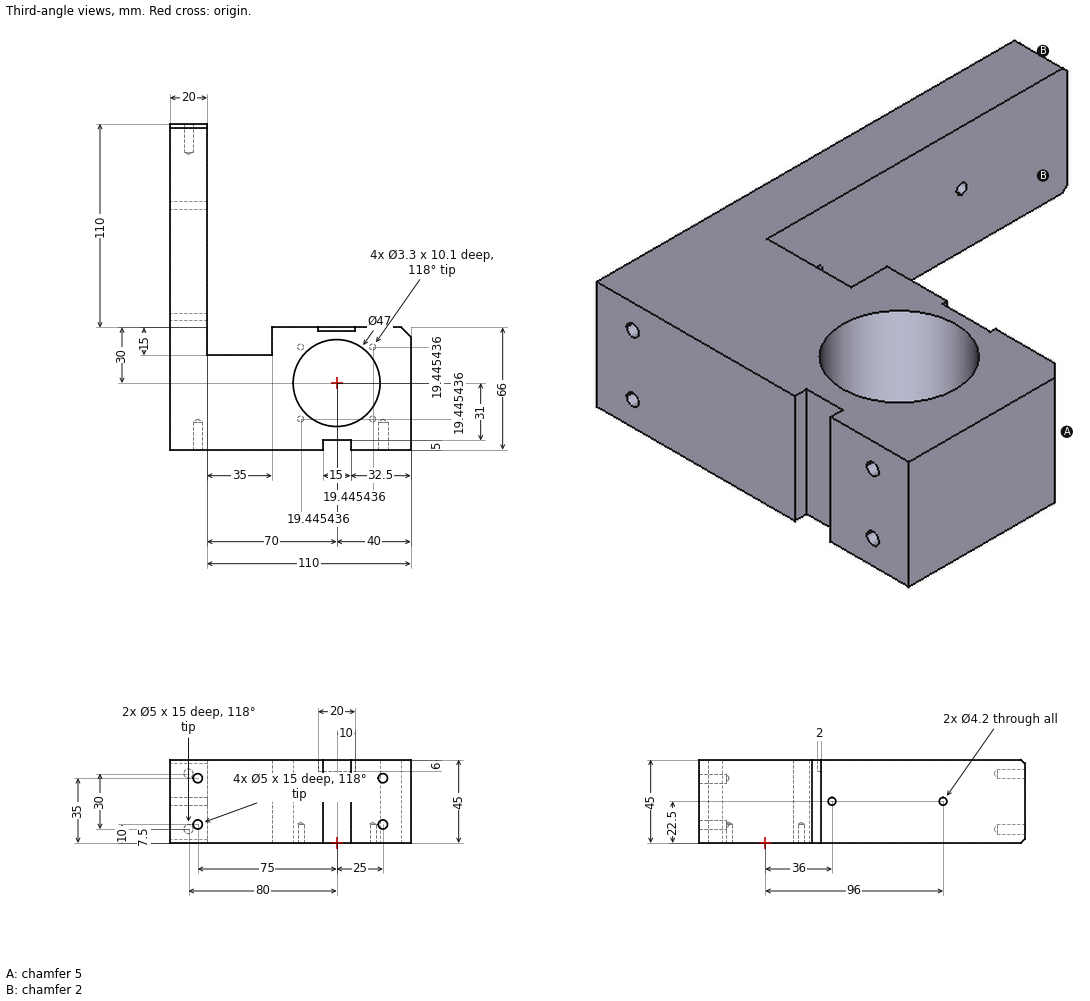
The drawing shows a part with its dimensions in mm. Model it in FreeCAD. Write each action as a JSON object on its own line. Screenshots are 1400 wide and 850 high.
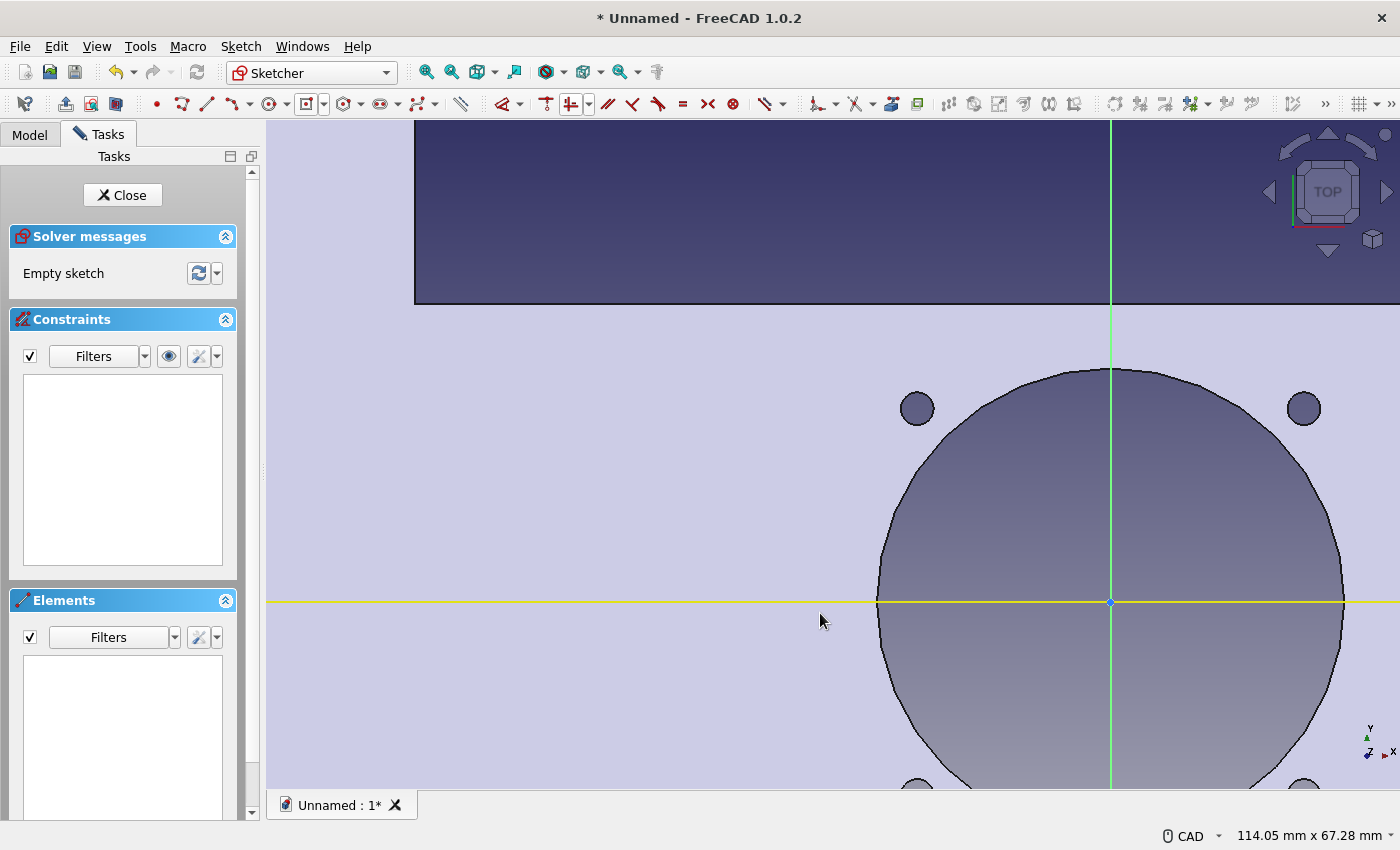
{"action": "left_click", "coordinate": [324, 104]}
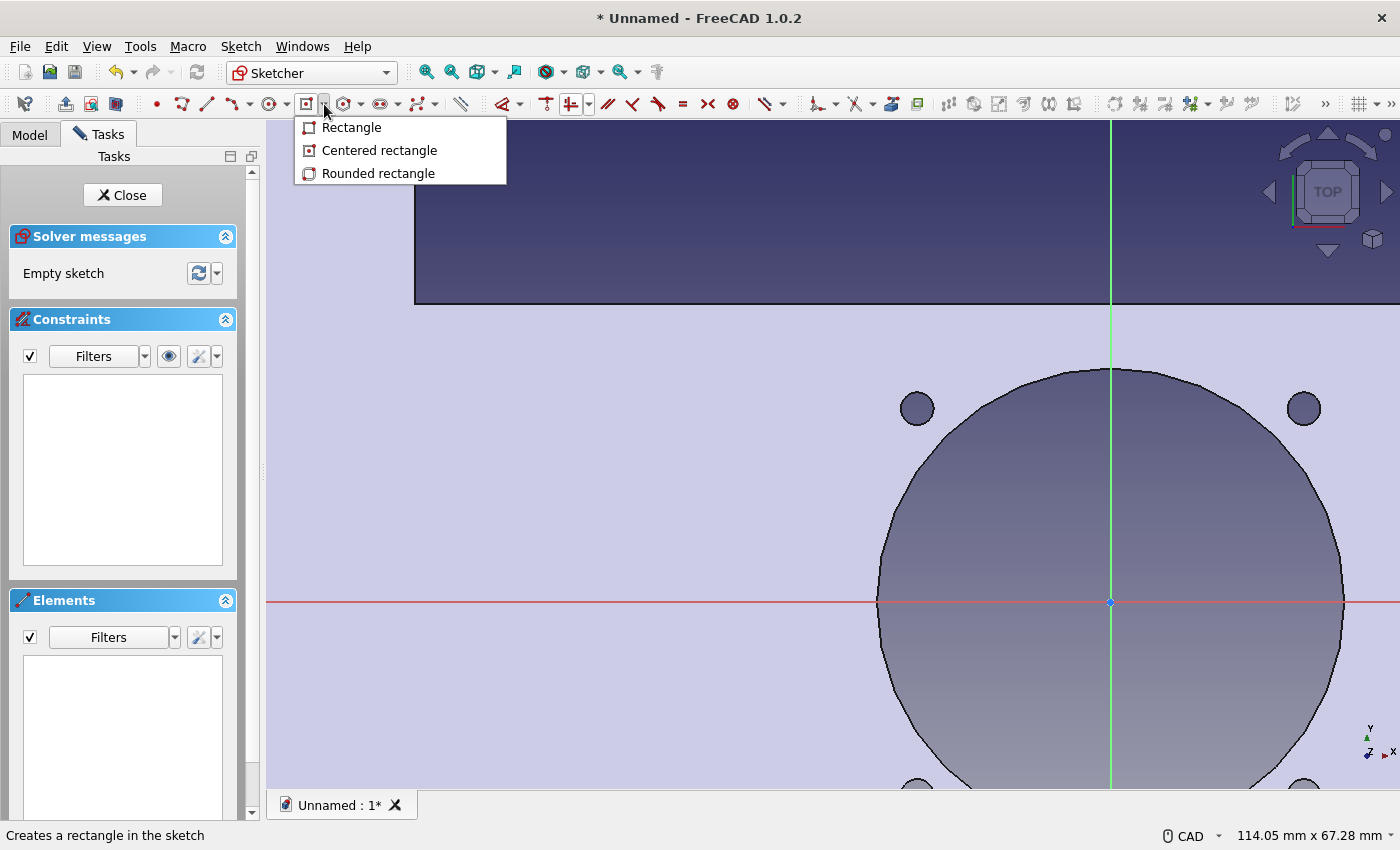
{"action": "left_click", "coordinate": [400, 128]}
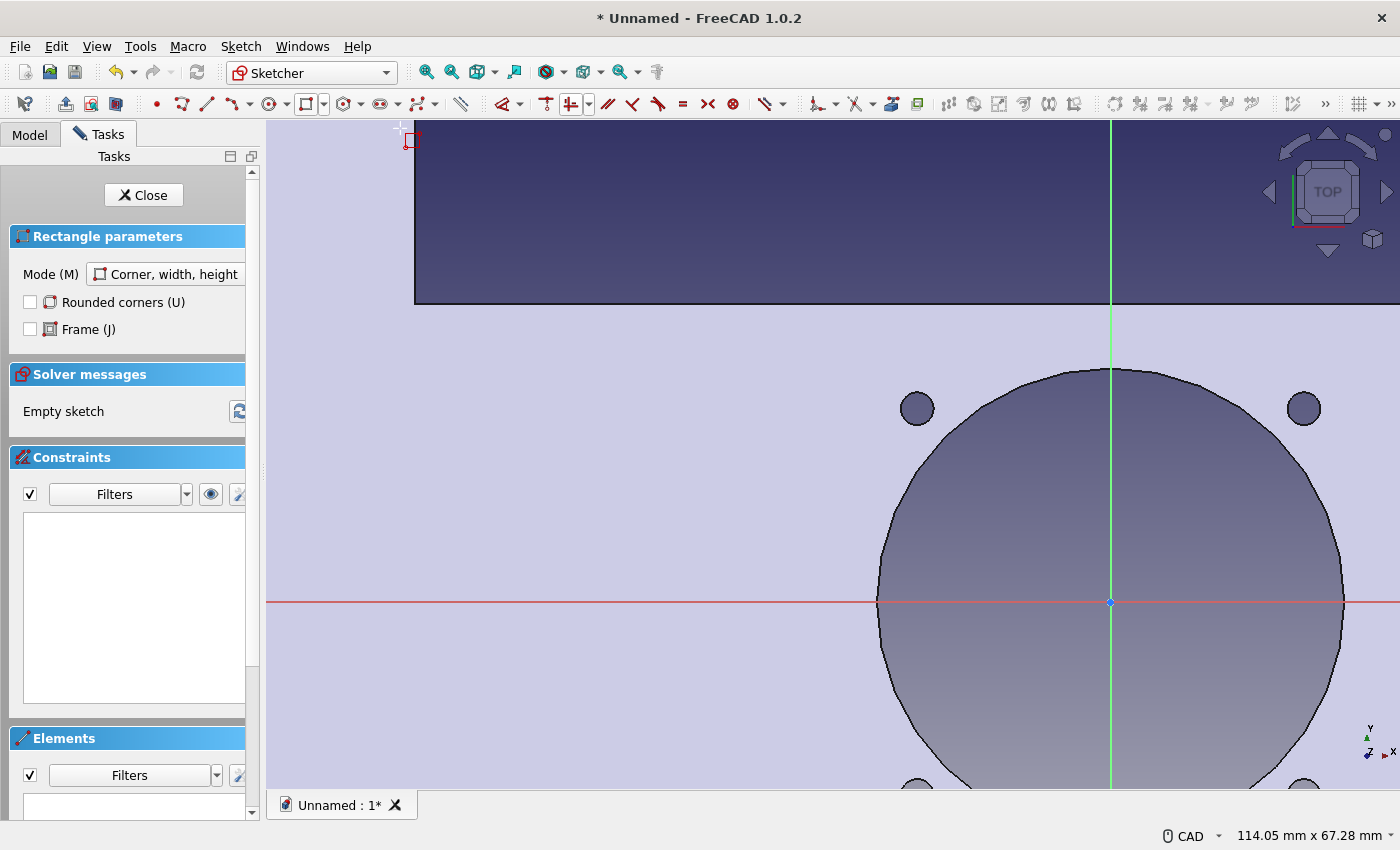
{"action": "left_click", "coordinate": [415, 304]}
{"action": "left_click", "coordinate": [763, 453]}
{"action": "key", "text": "Escape"}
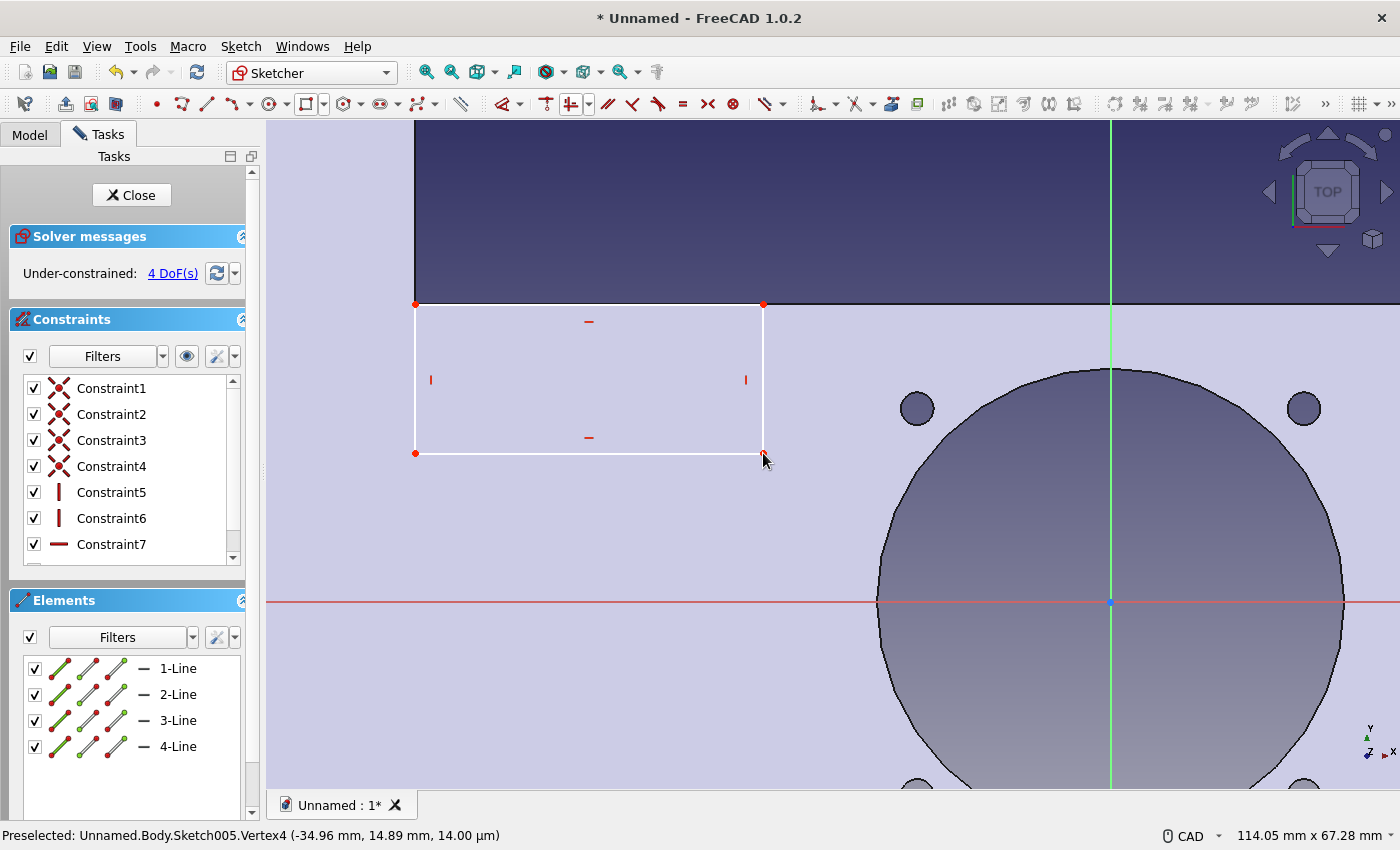
{"action": "left_click", "coordinate": [502, 104]}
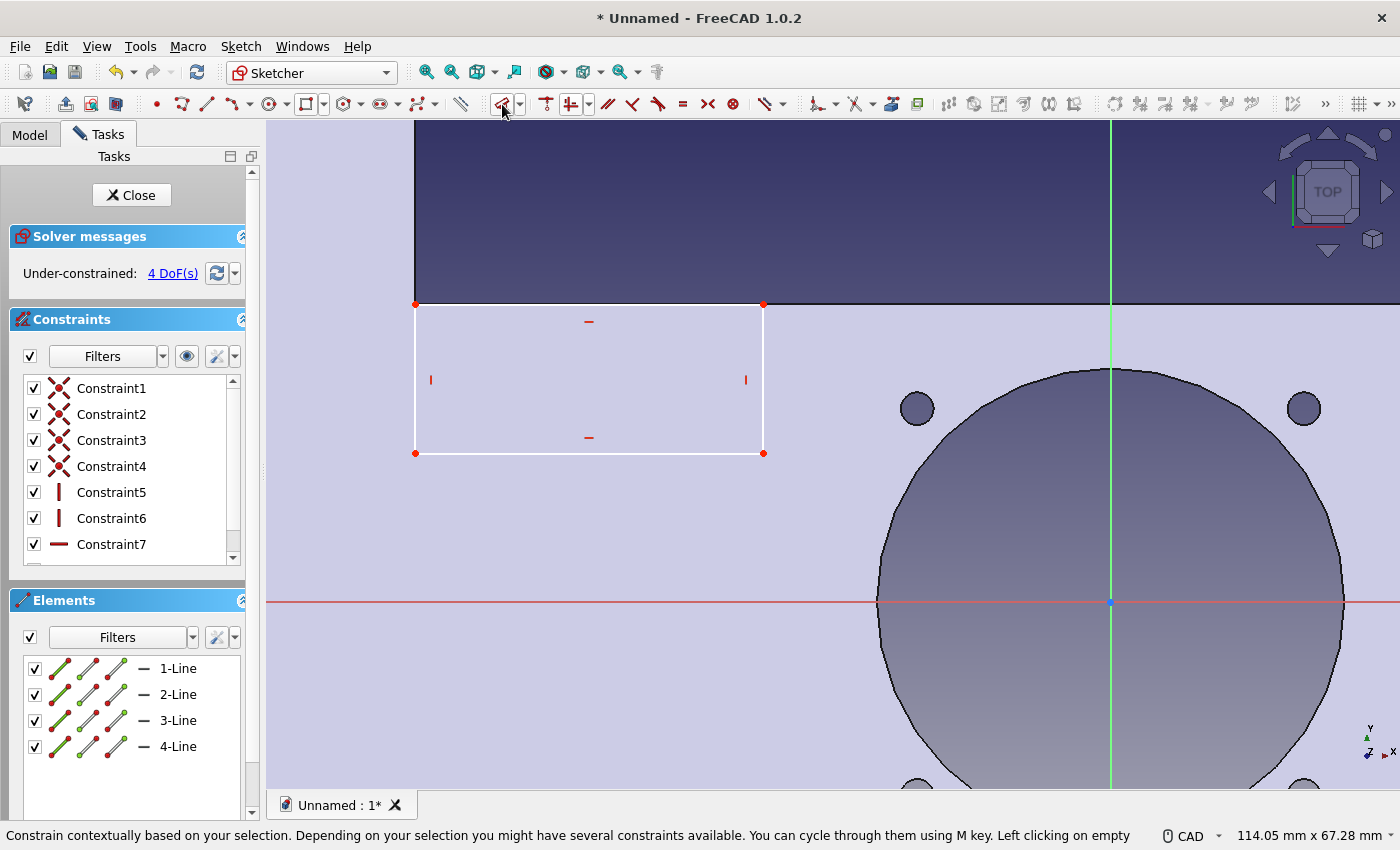
{"action": "left_click", "coordinate": [415, 350]}
{"action": "left_click", "coordinate": [381, 379]}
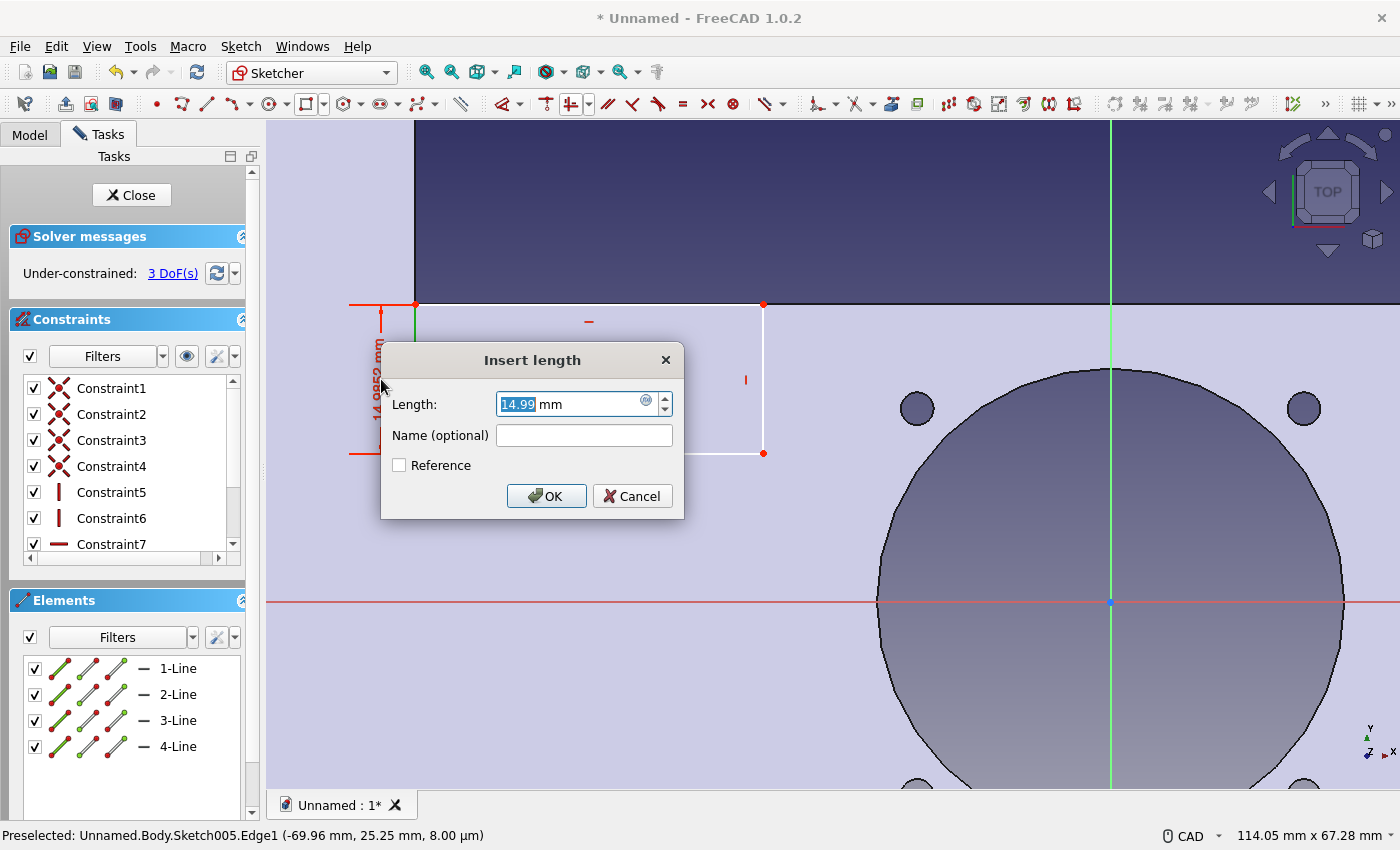
{"action": "type", "text": "15"}
{"action": "key", "text": "Return"}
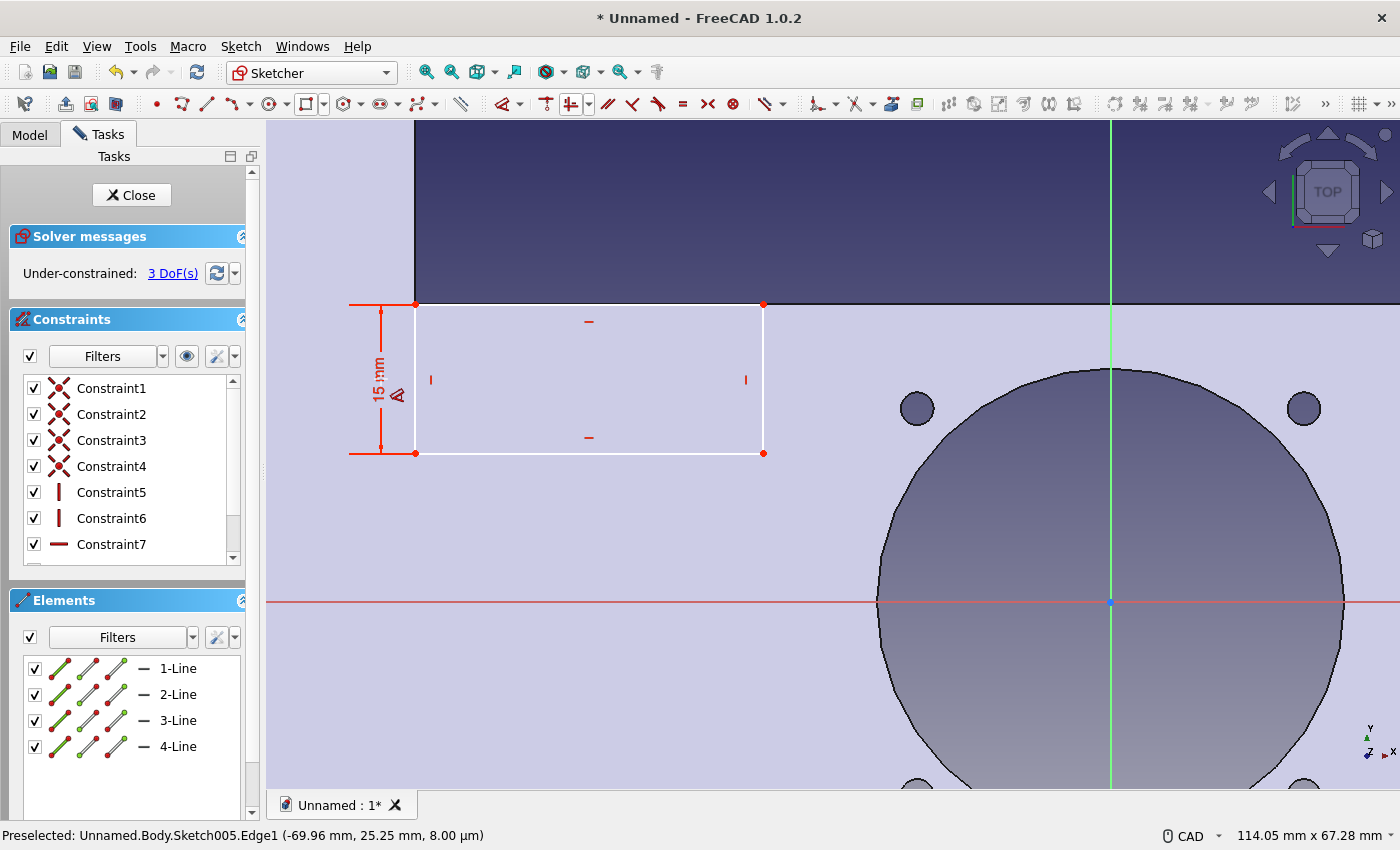
{"action": "left_click", "coordinate": [519, 454]}
{"action": "left_click", "coordinate": [589, 488]}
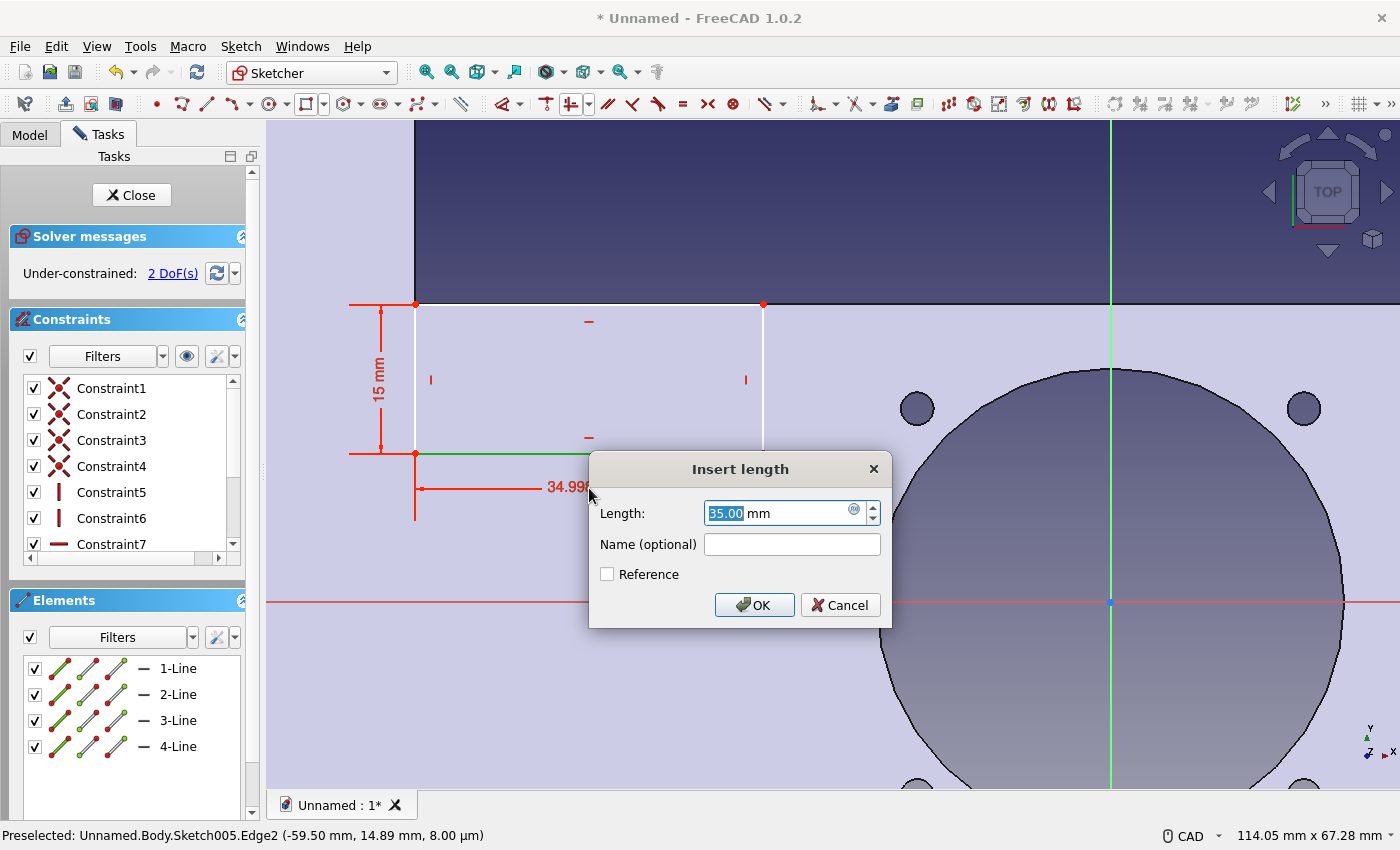
{"action": "type", "text": "35"}
{"action": "key", "text": "Return"}